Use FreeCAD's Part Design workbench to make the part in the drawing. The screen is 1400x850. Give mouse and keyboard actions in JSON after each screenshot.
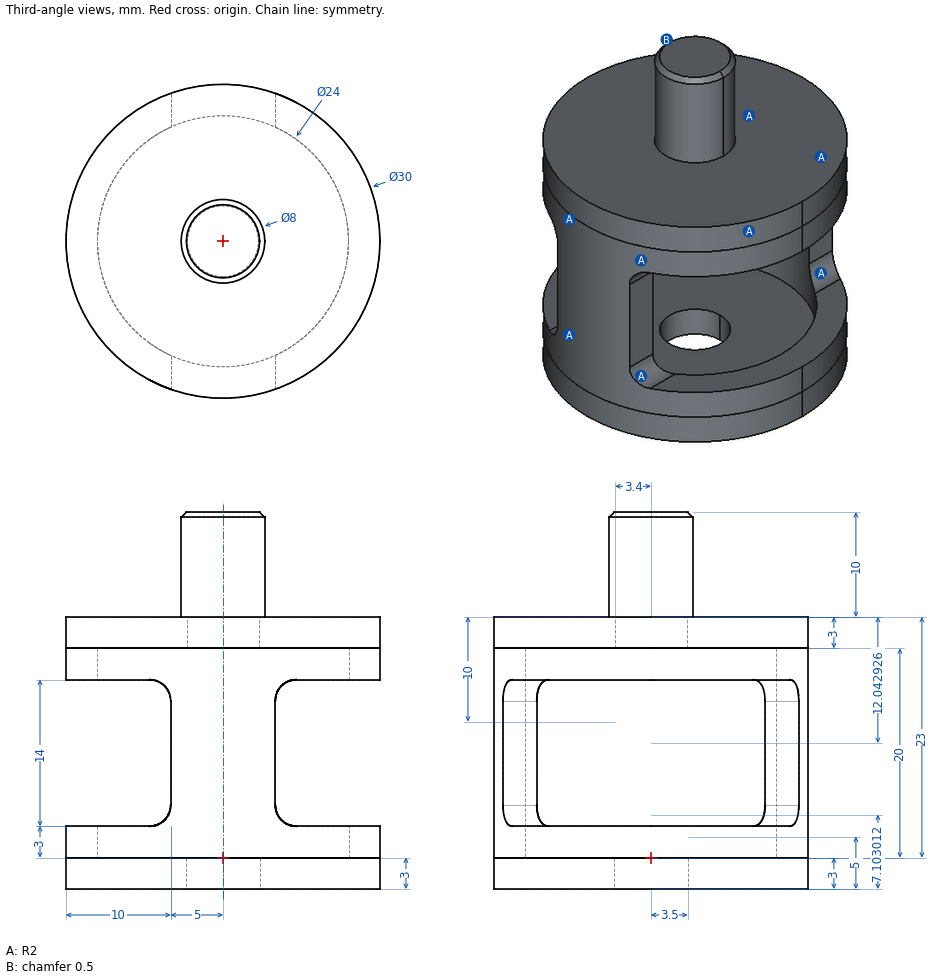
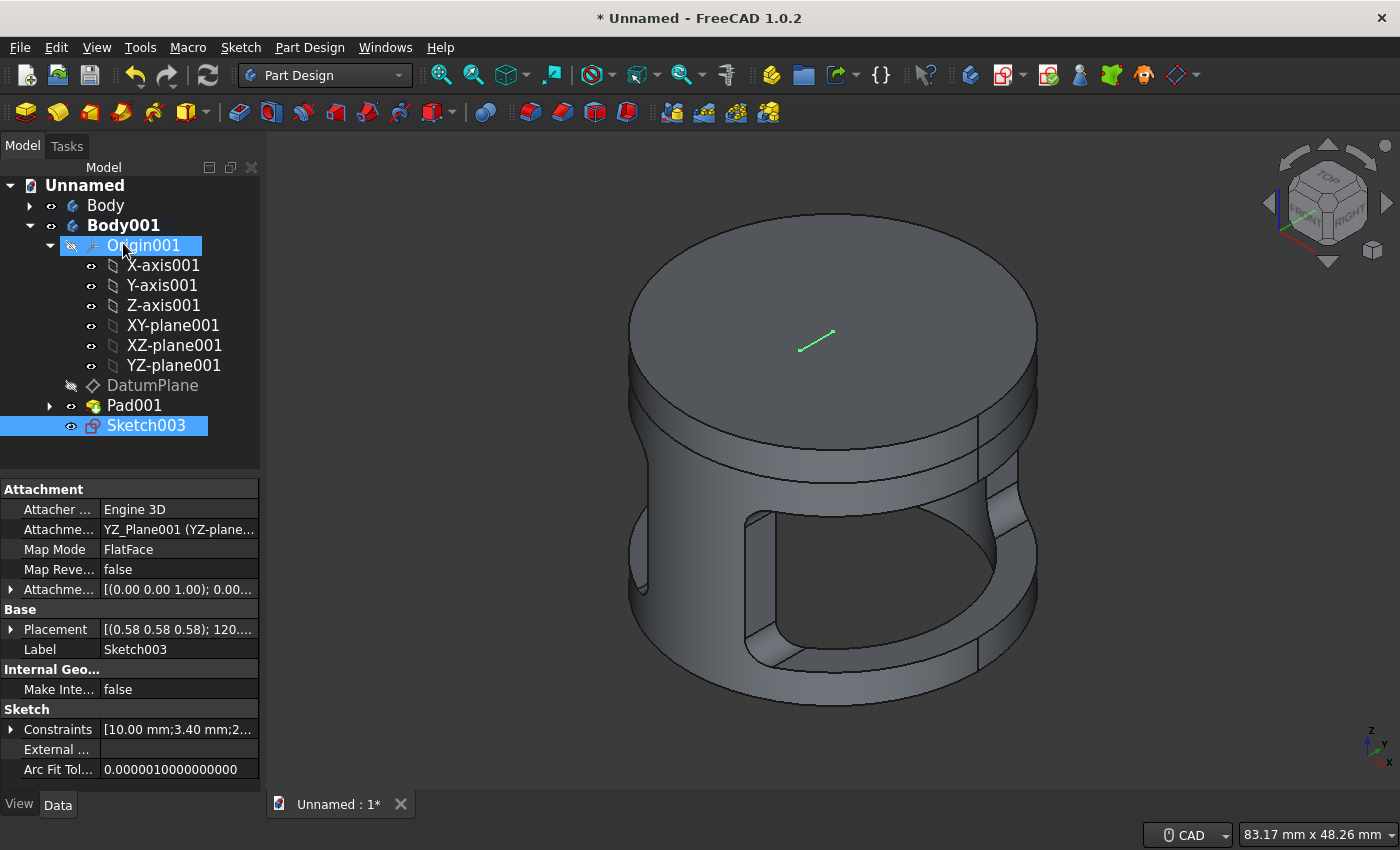
{"action": "left_click", "coordinate": [304, 112]}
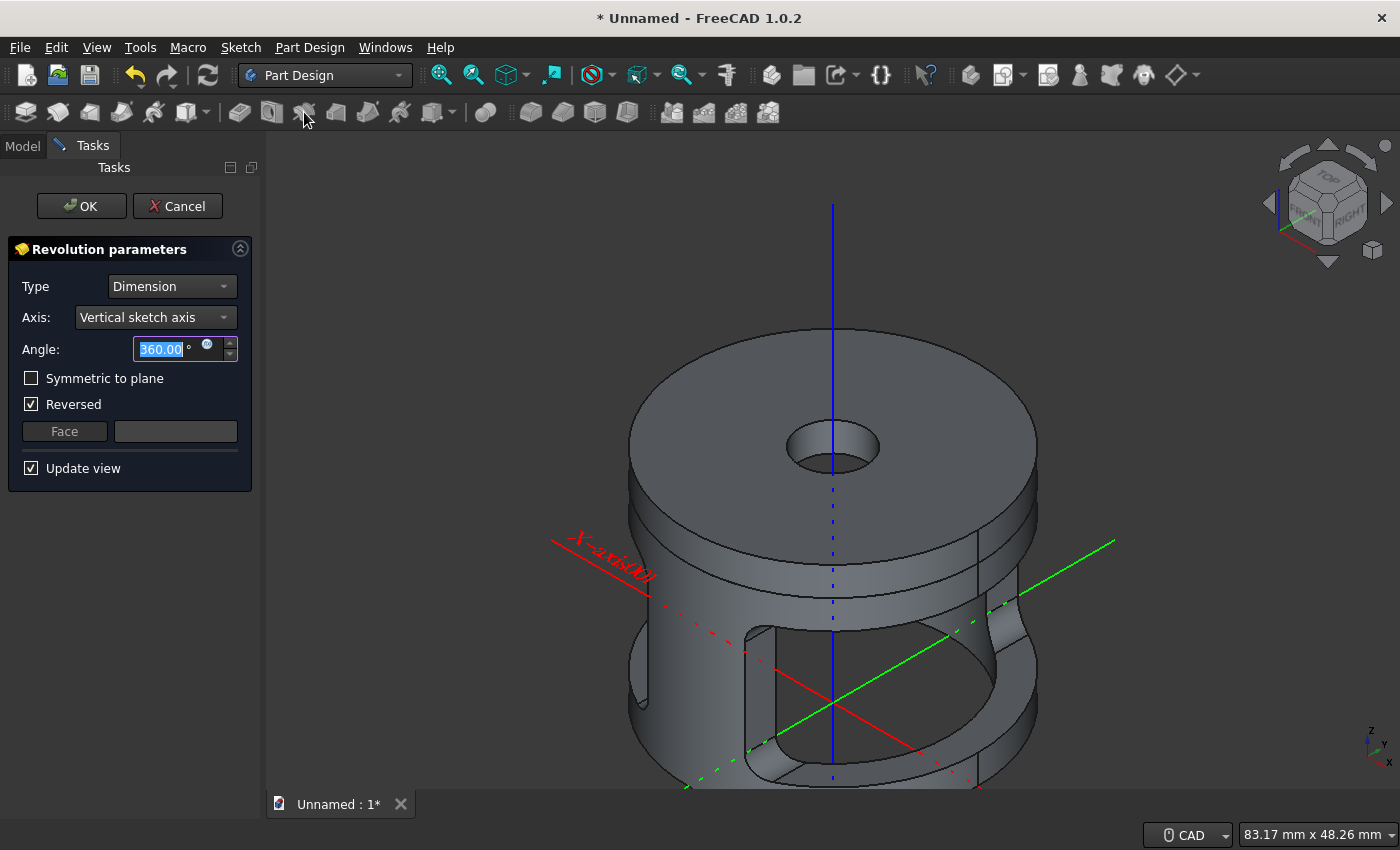
{"action": "left_click", "coordinate": [82, 206]}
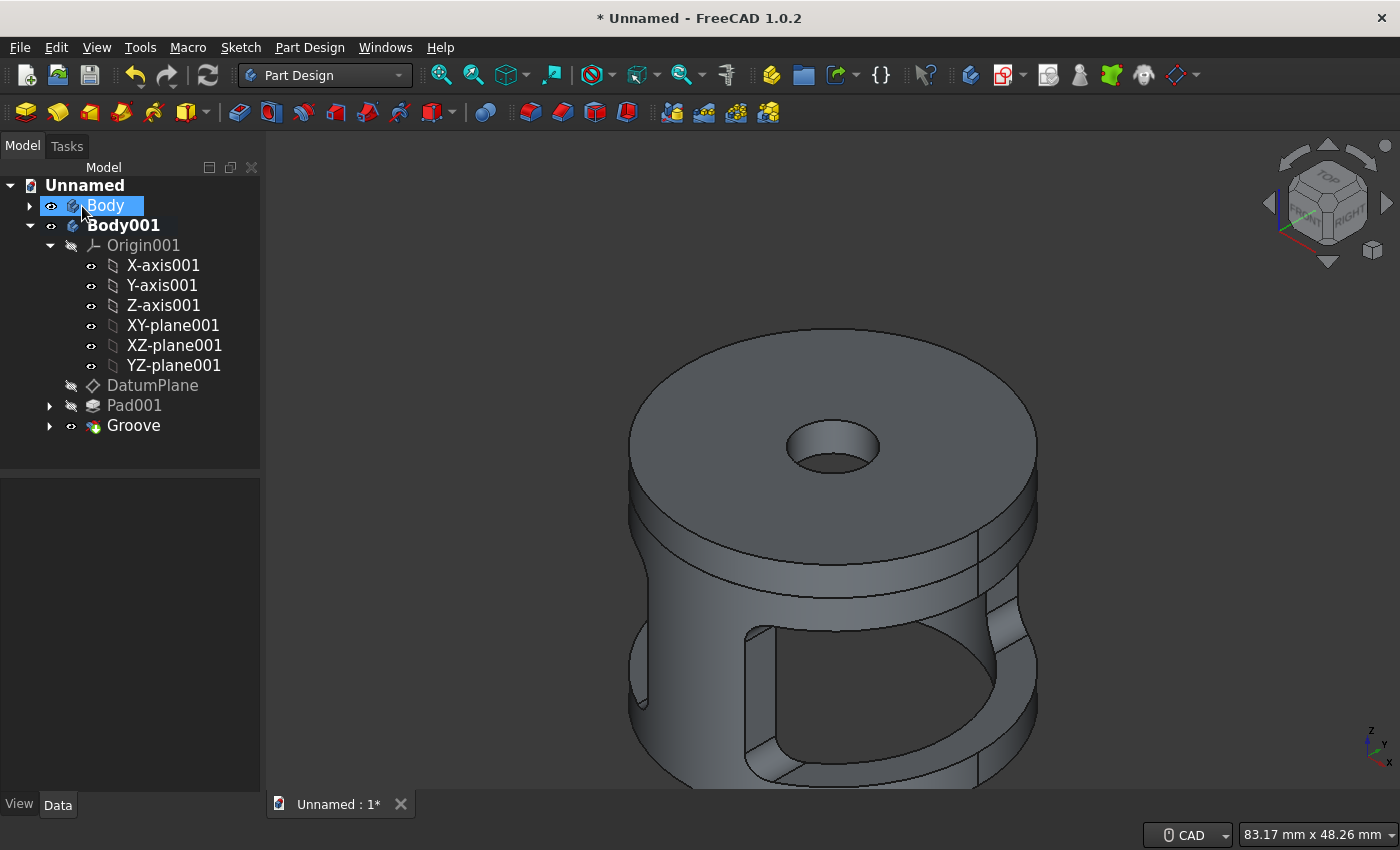
{"action": "left_click", "coordinate": [792, 517]}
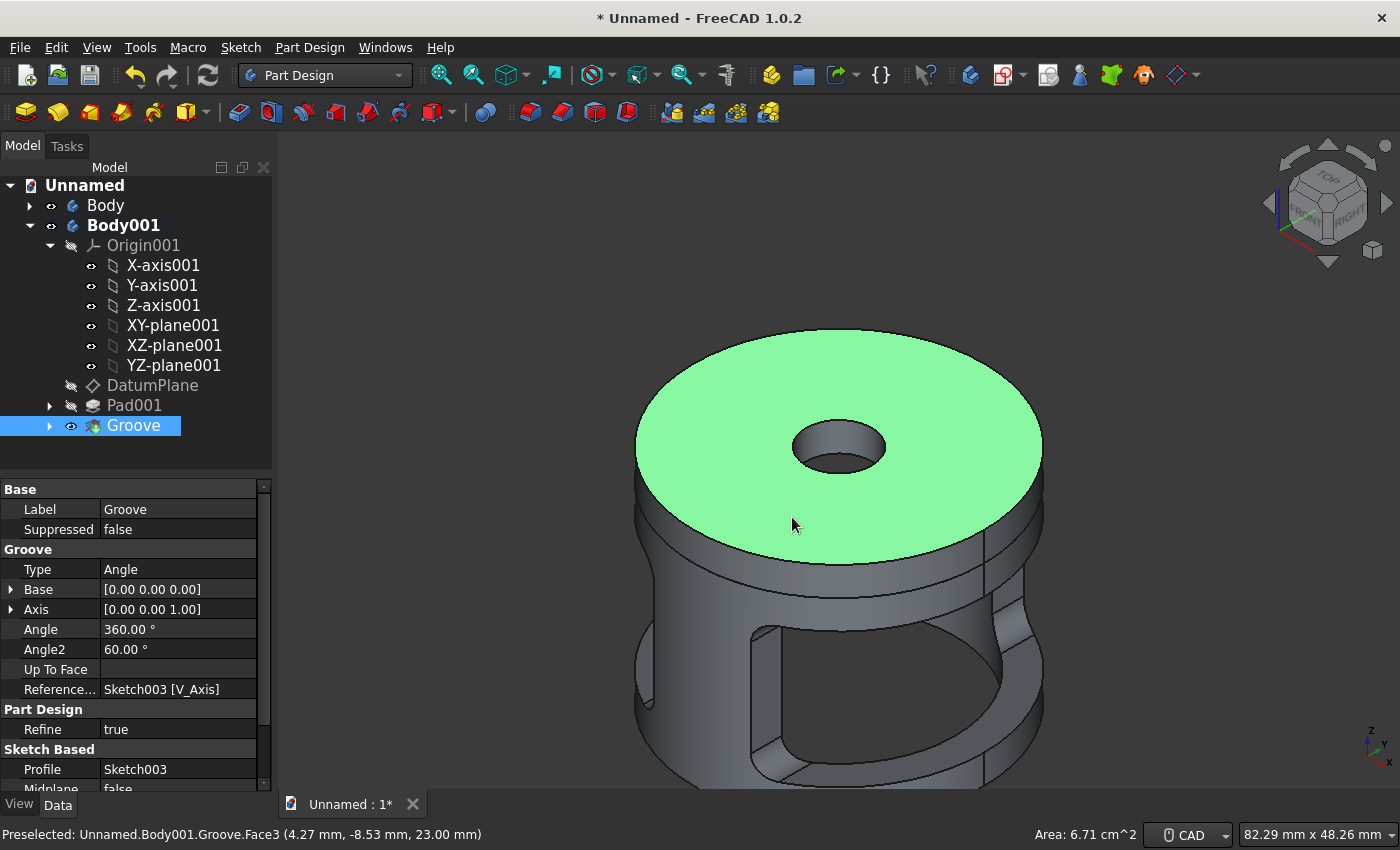
{"action": "left_click", "coordinate": [1004, 76]}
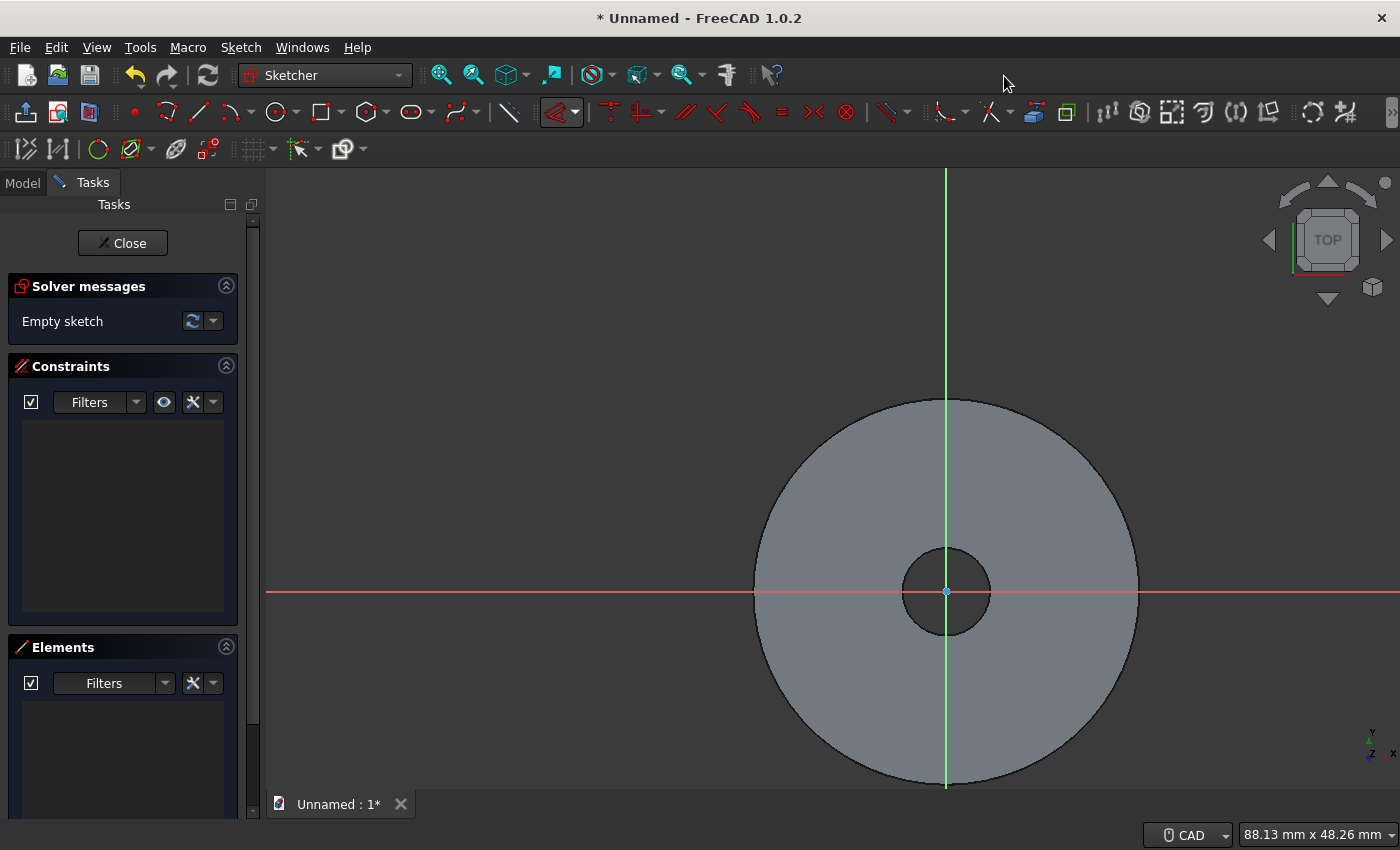
{"action": "scroll", "coordinate": [1006, 629], "scroll_direction": "up", "scroll_amount": 7}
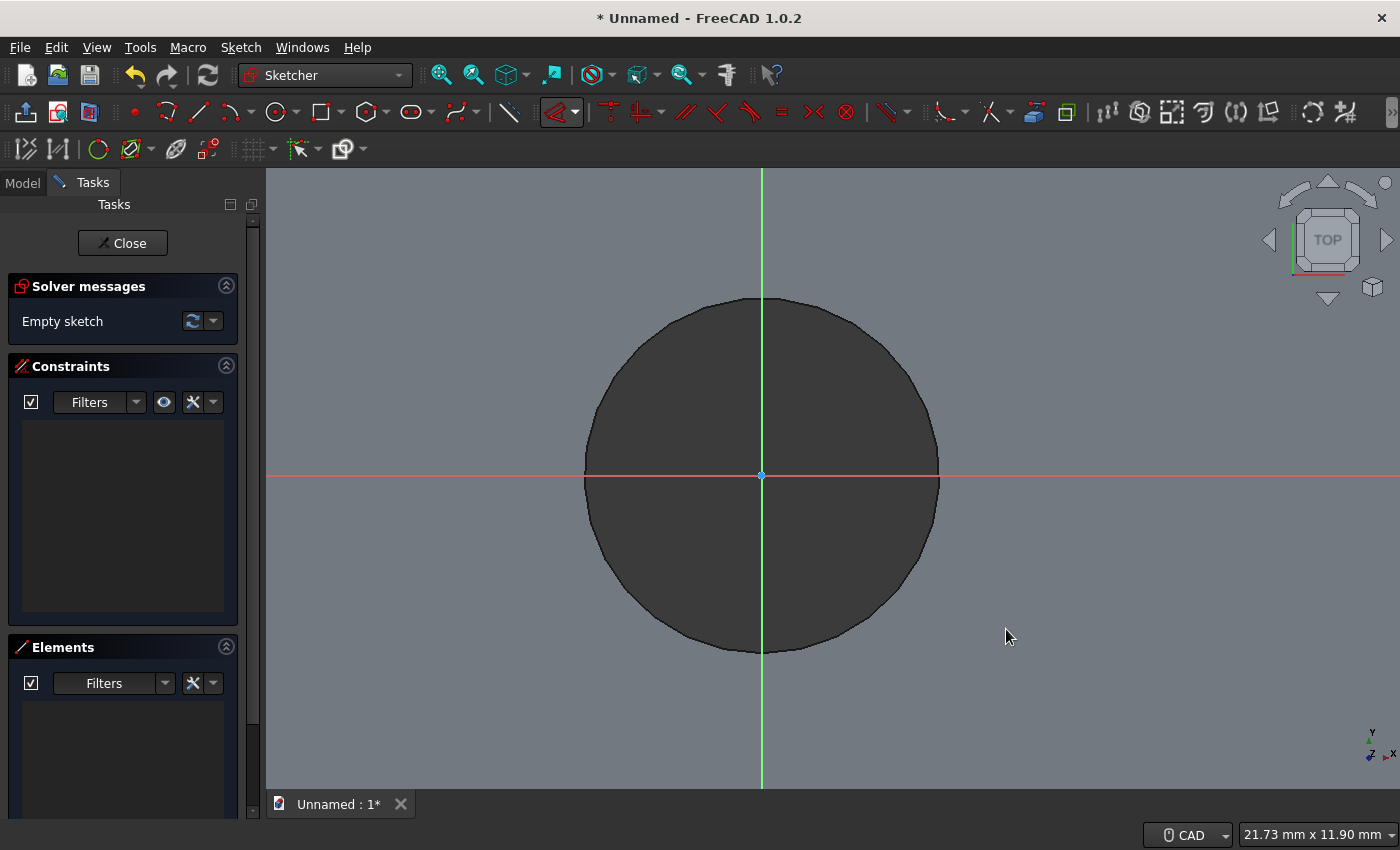
{"action": "key", "text": "g c"}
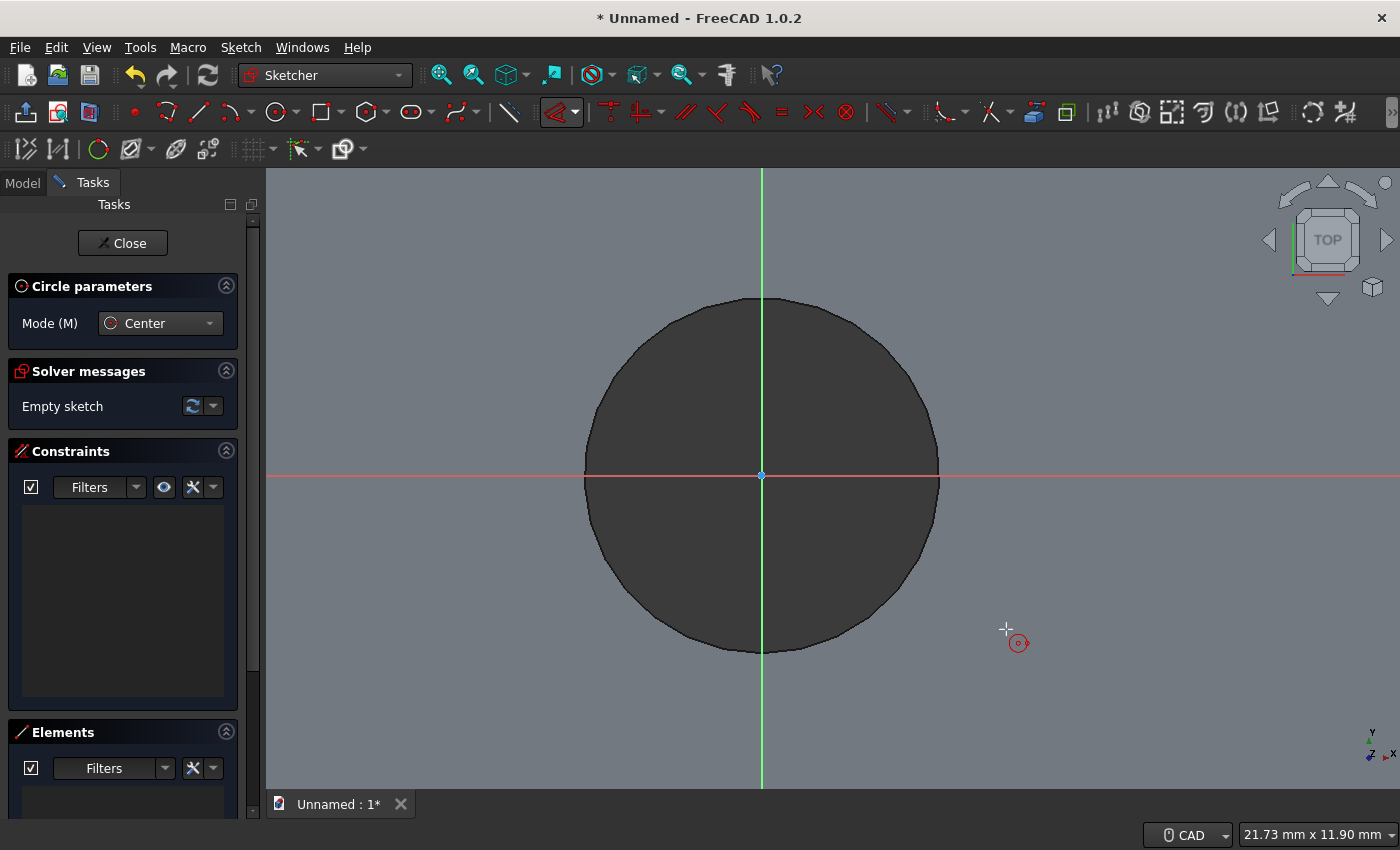
{"action": "left_click", "coordinate": [762, 476]}
{"action": "left_click", "coordinate": [909, 328]}
{"action": "key", "text": "Escape"}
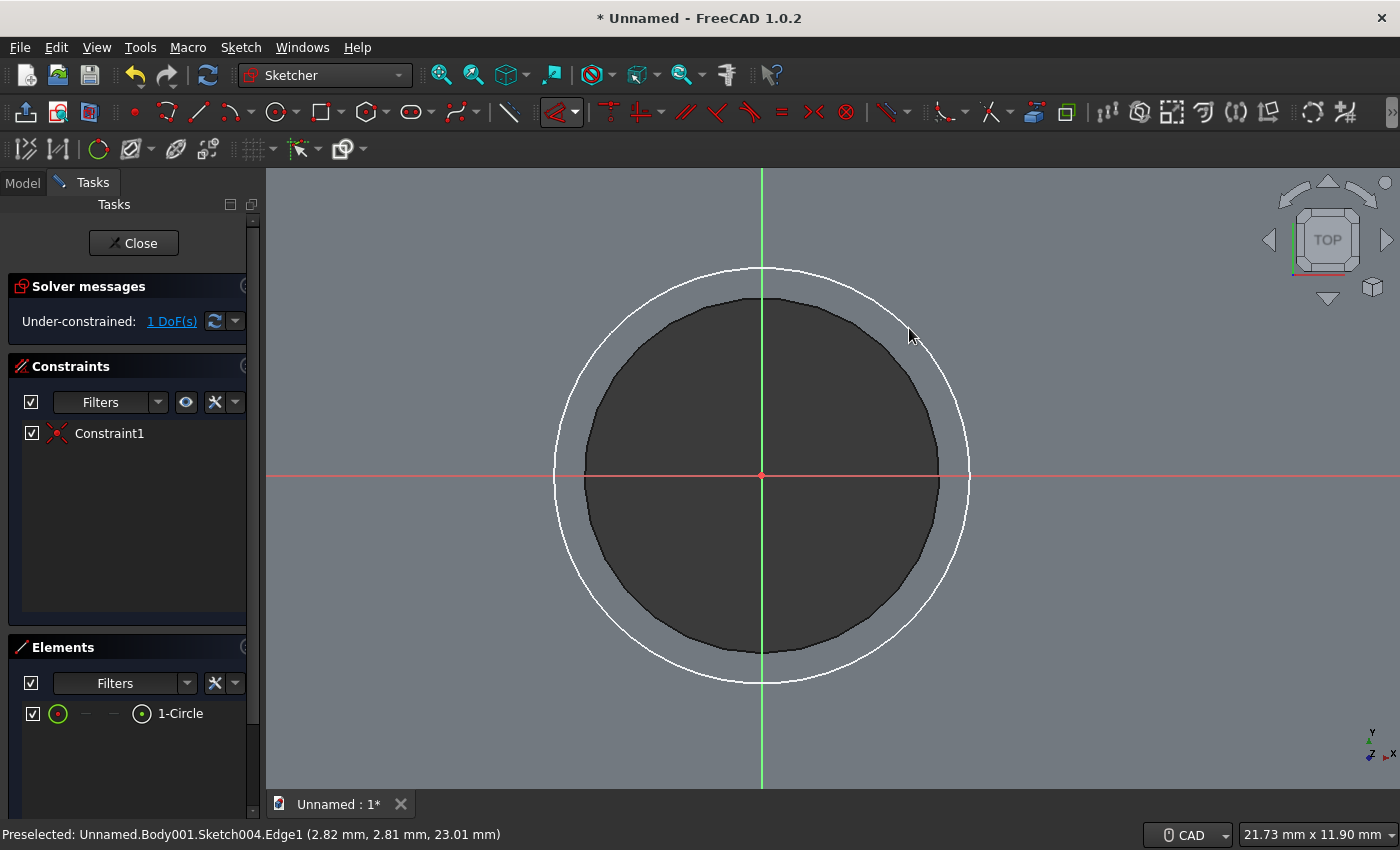
{"action": "left_click", "coordinate": [908, 328]}